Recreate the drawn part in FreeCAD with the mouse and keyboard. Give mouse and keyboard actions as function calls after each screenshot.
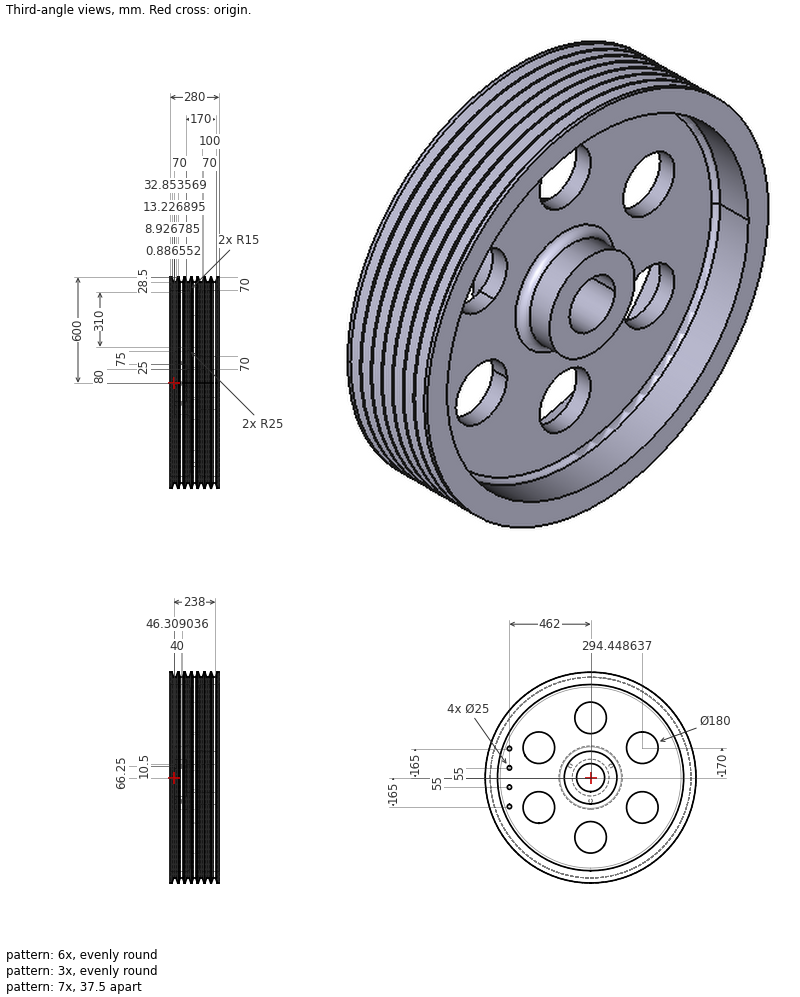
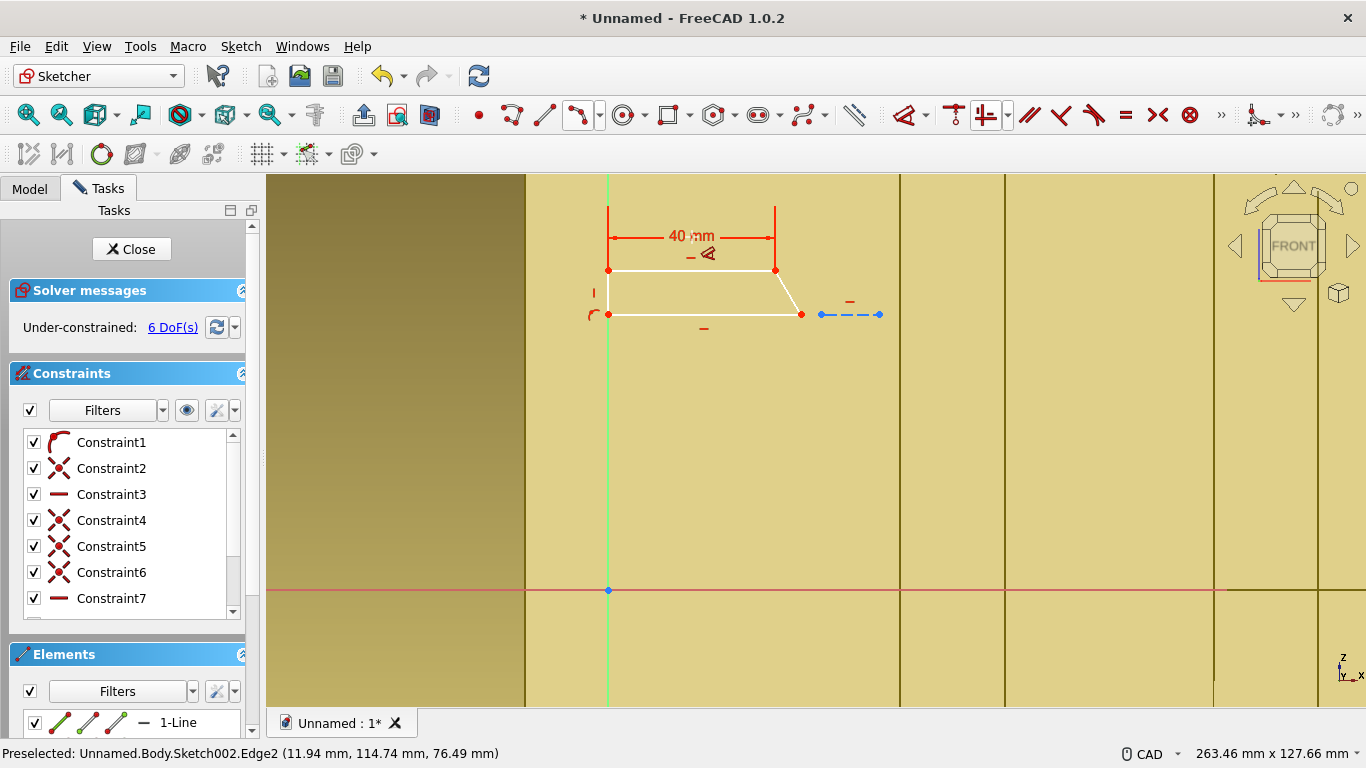
click(608, 302)
click(574, 293)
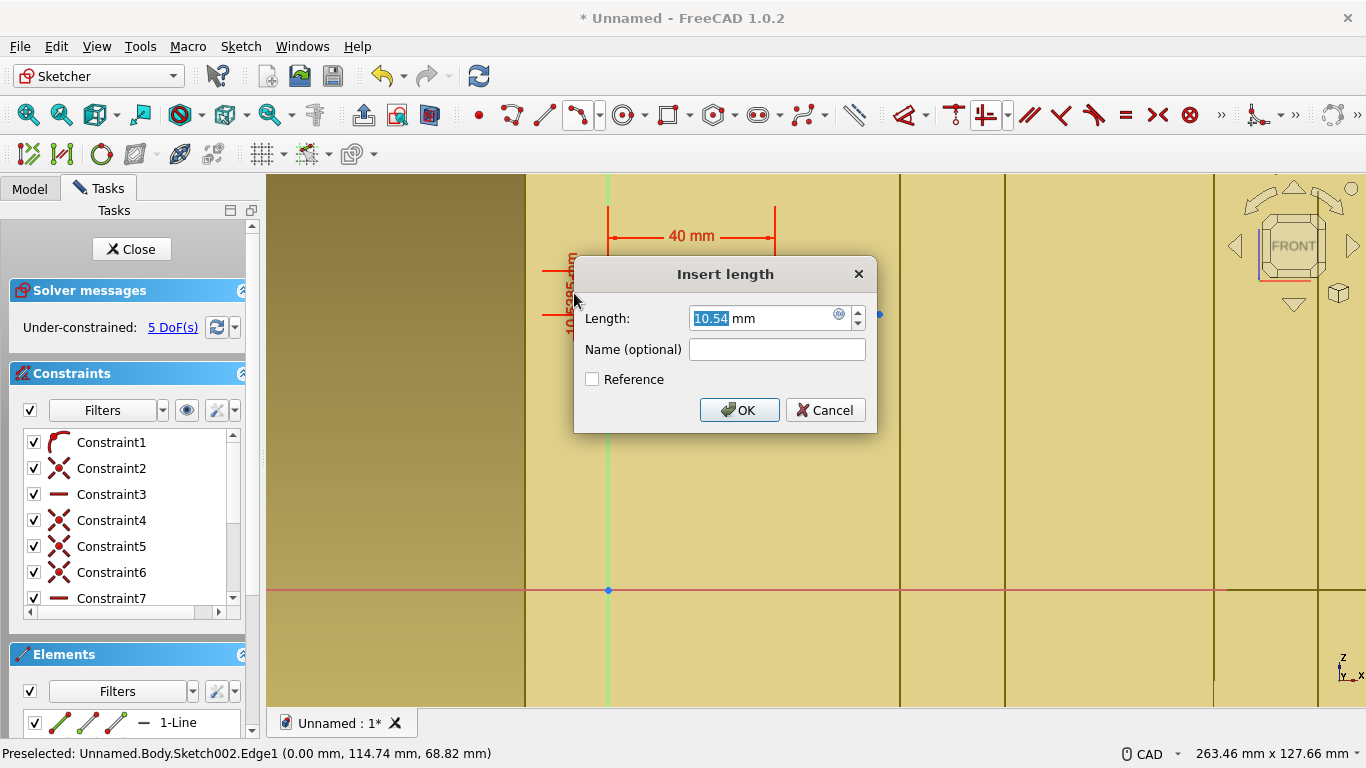
text(10.5)
key(Return)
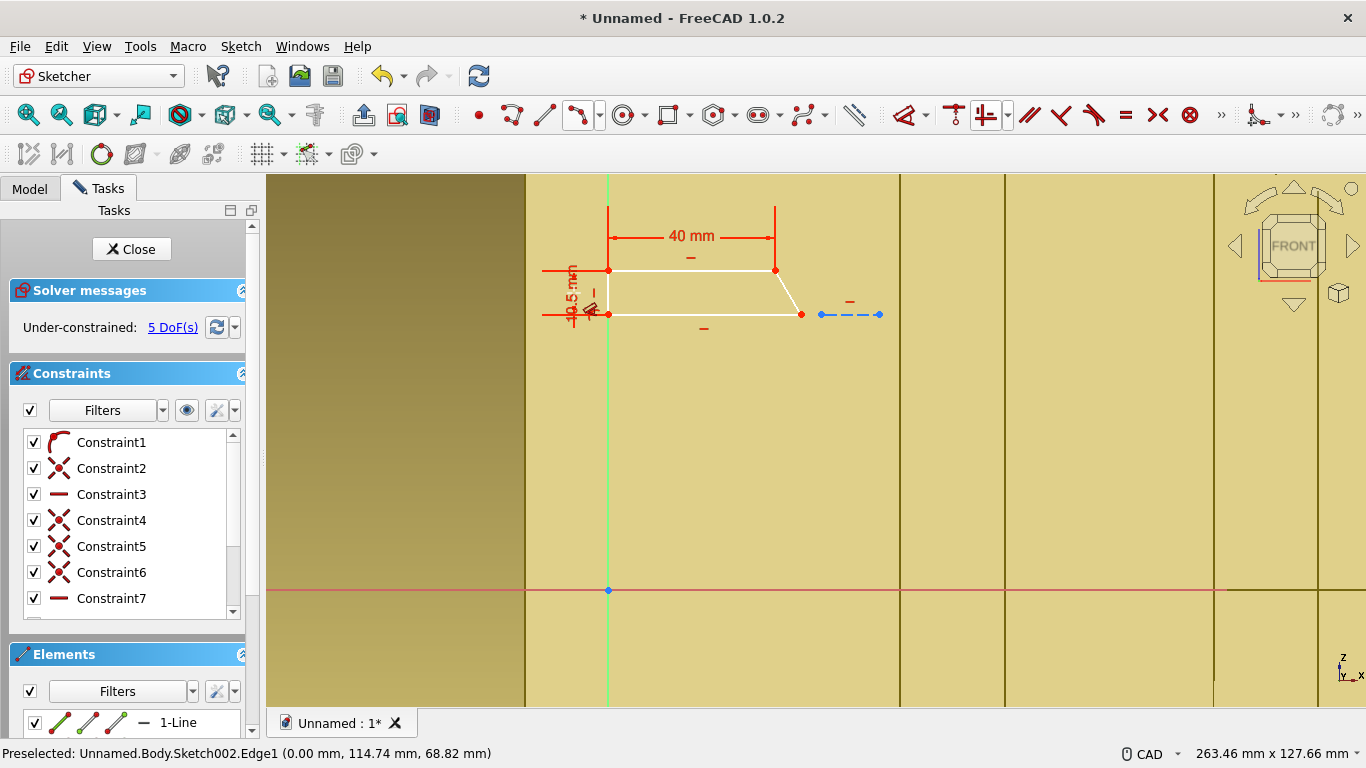
click(608, 315)
click(574, 453)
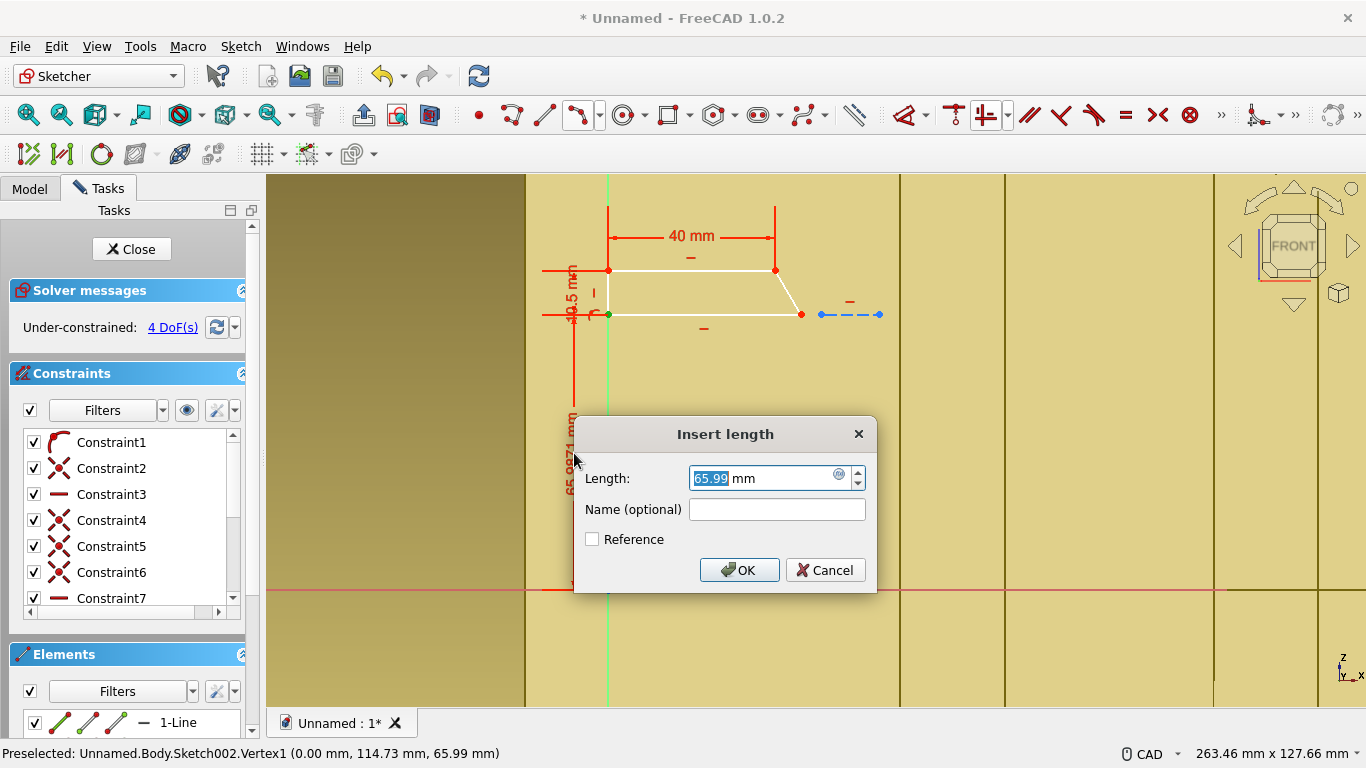
text(66.25)
key(Return)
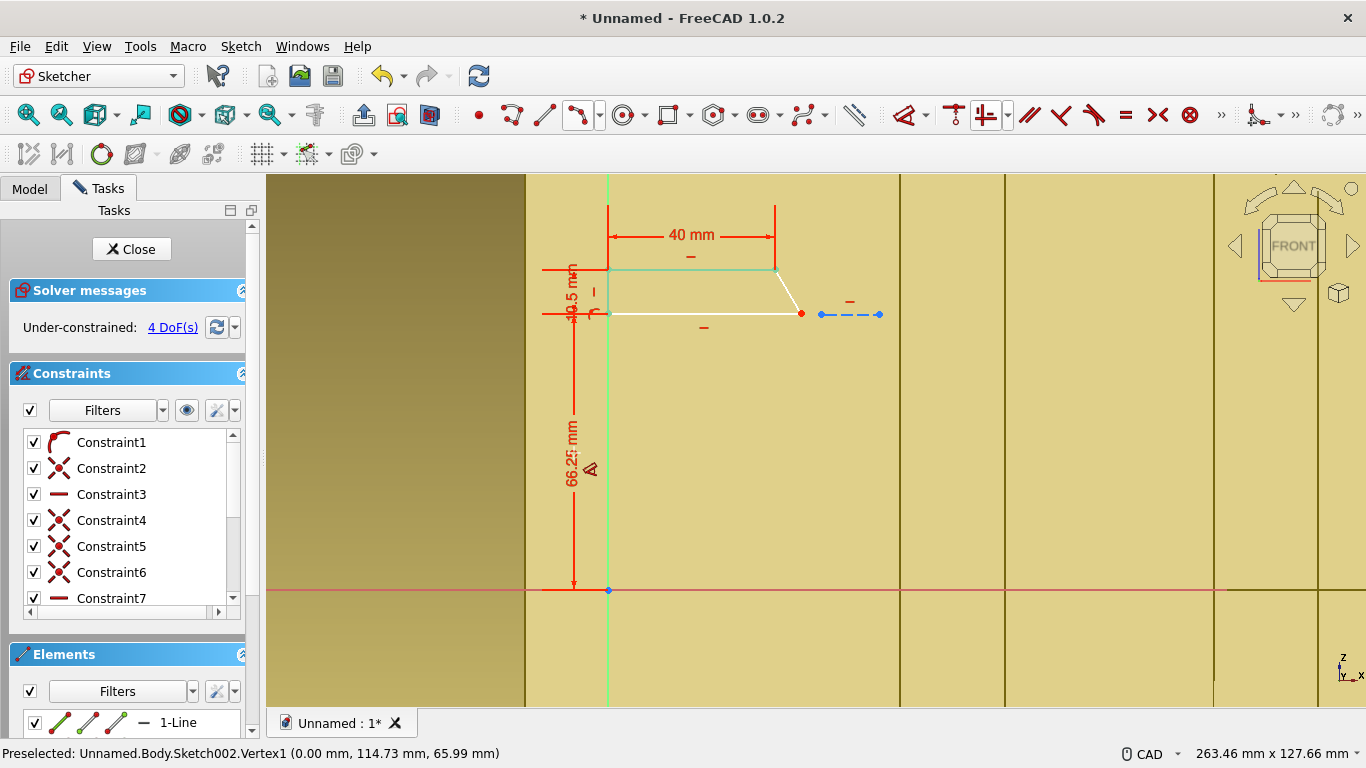
click(821, 315)
click(574, 389)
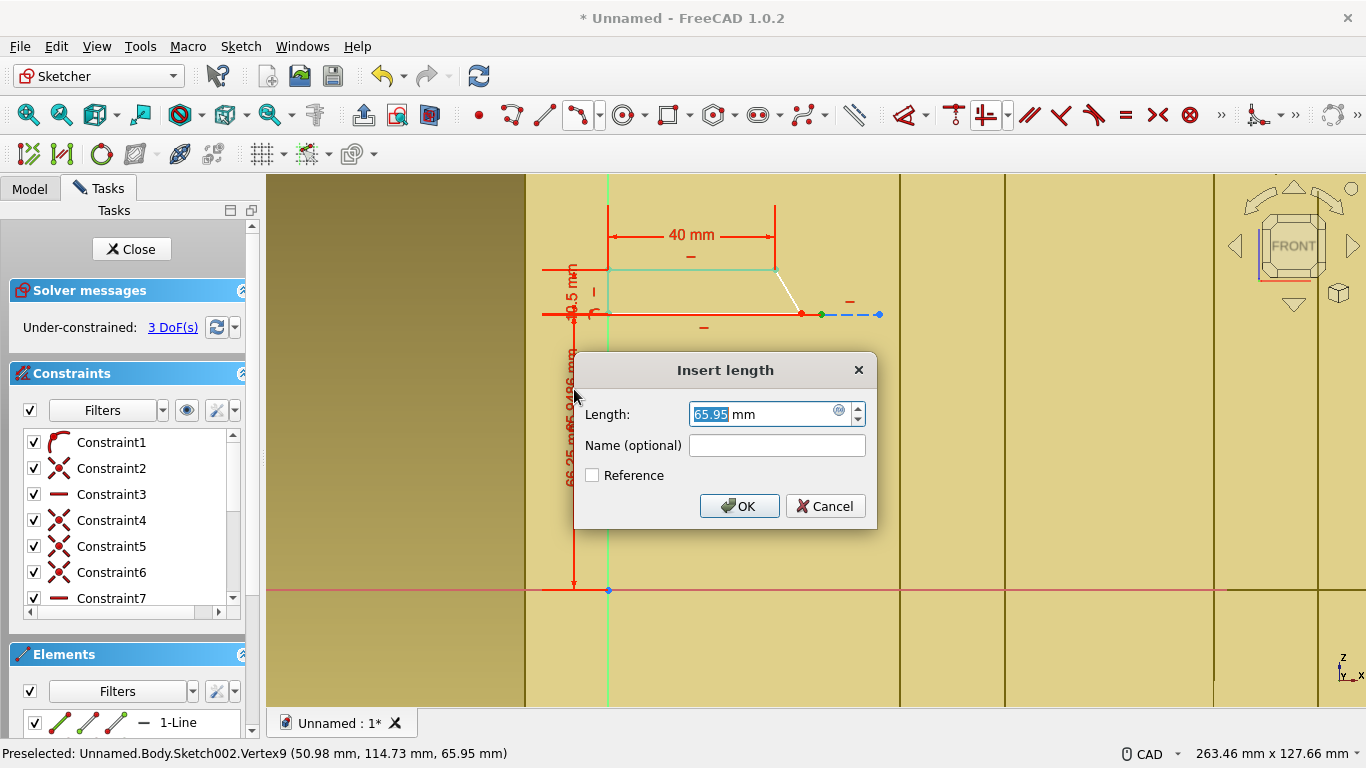
text(66.25)
key(Return)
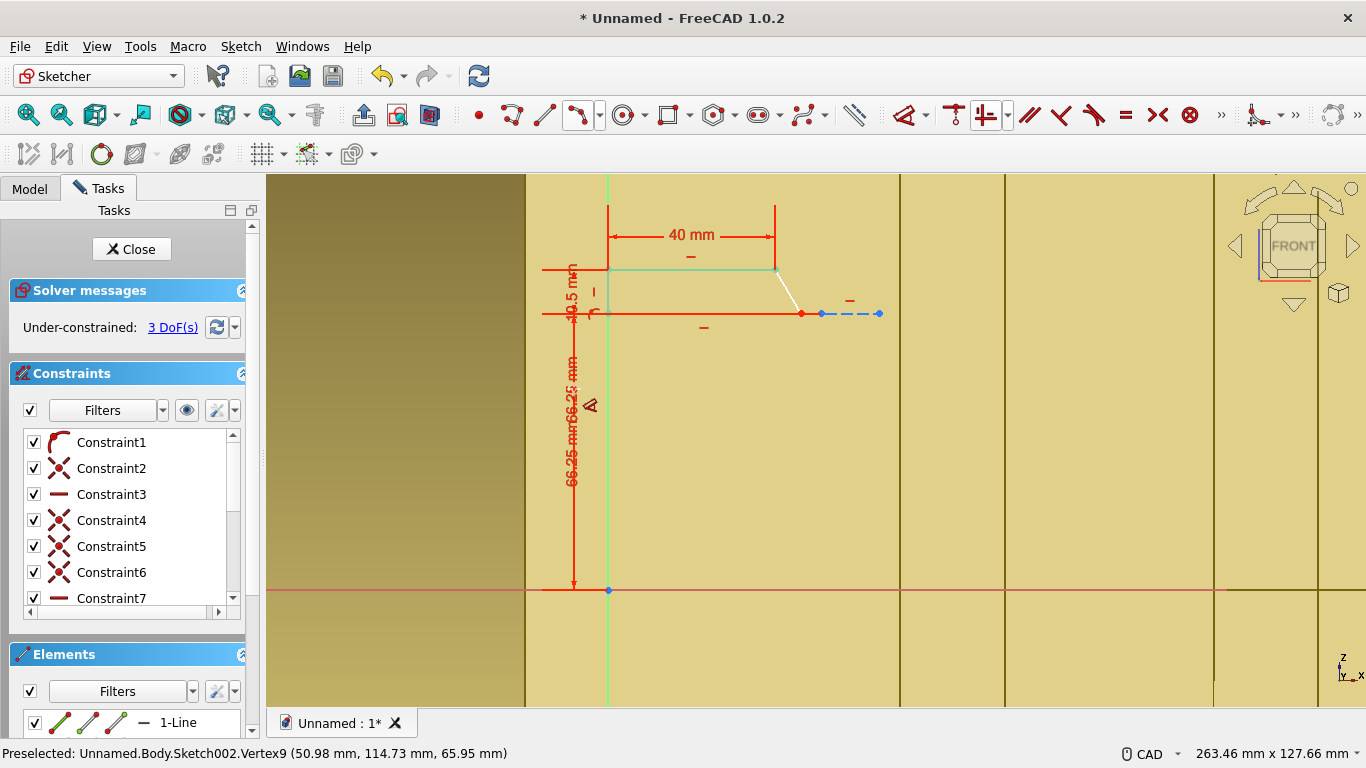
click(743, 314)
click(705, 348)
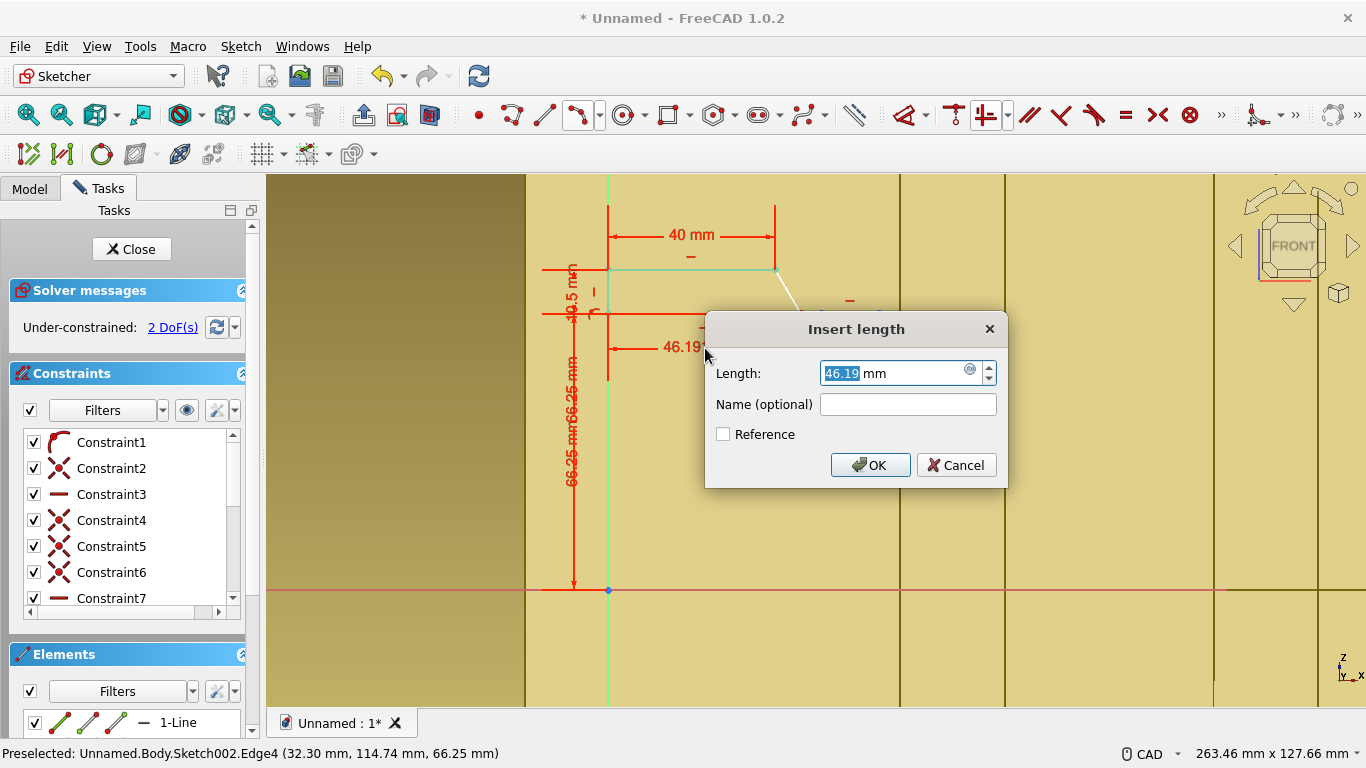
text(46.309036)
key(Return)
key(Escape)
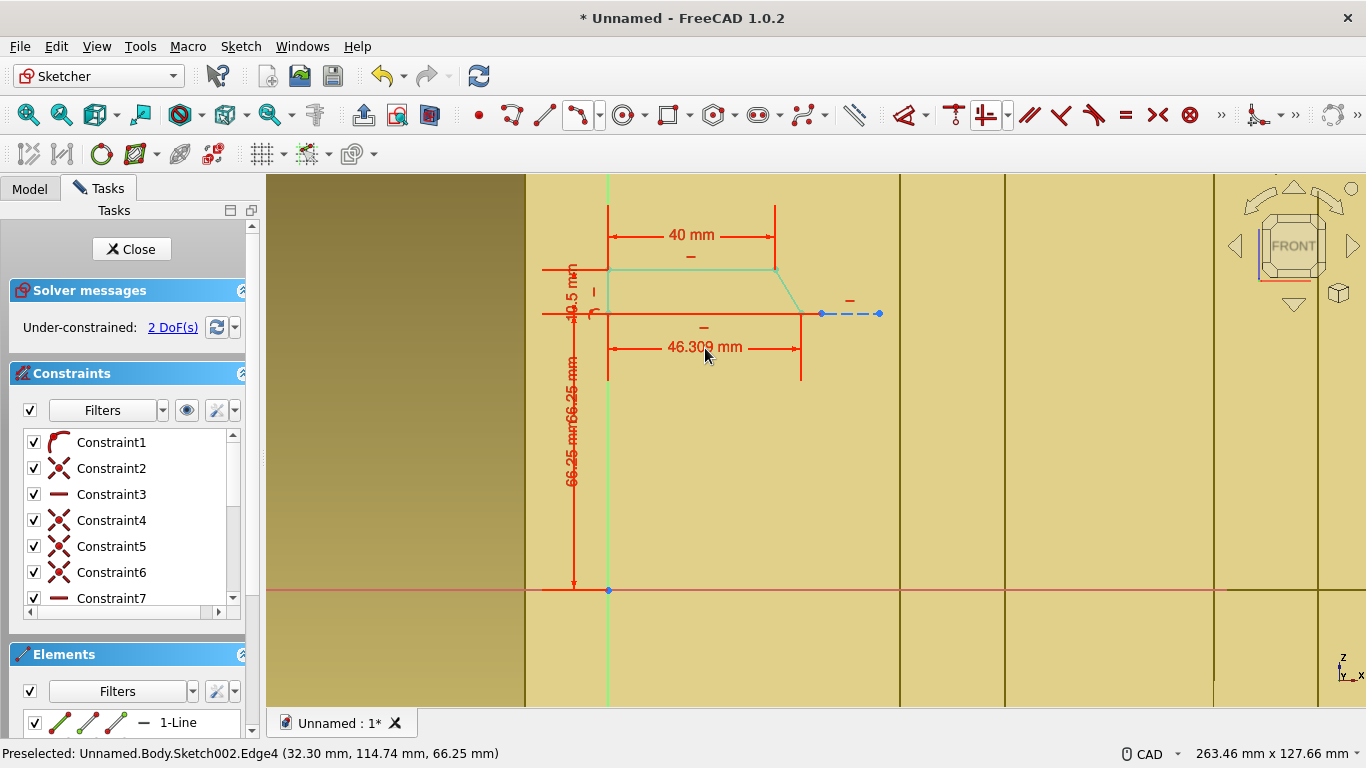
click(132, 249)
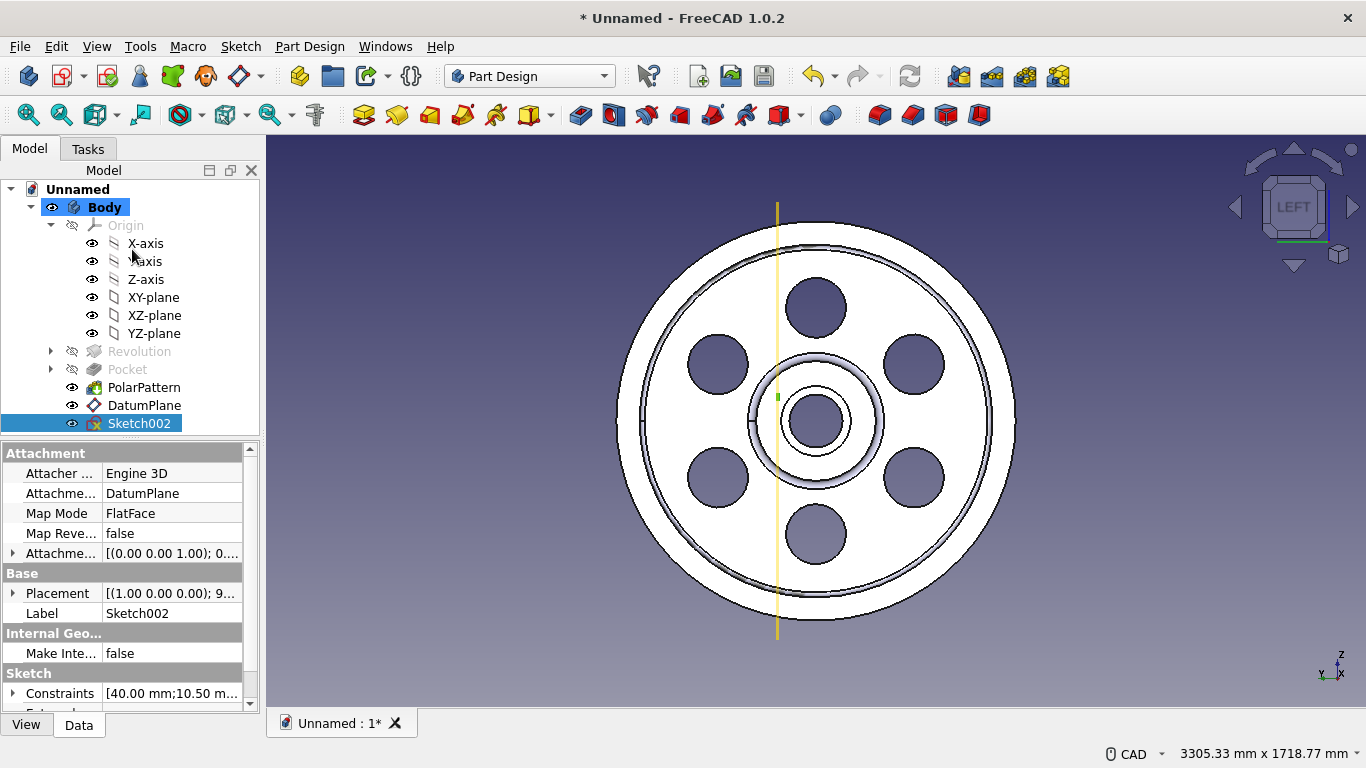
click(647, 116)